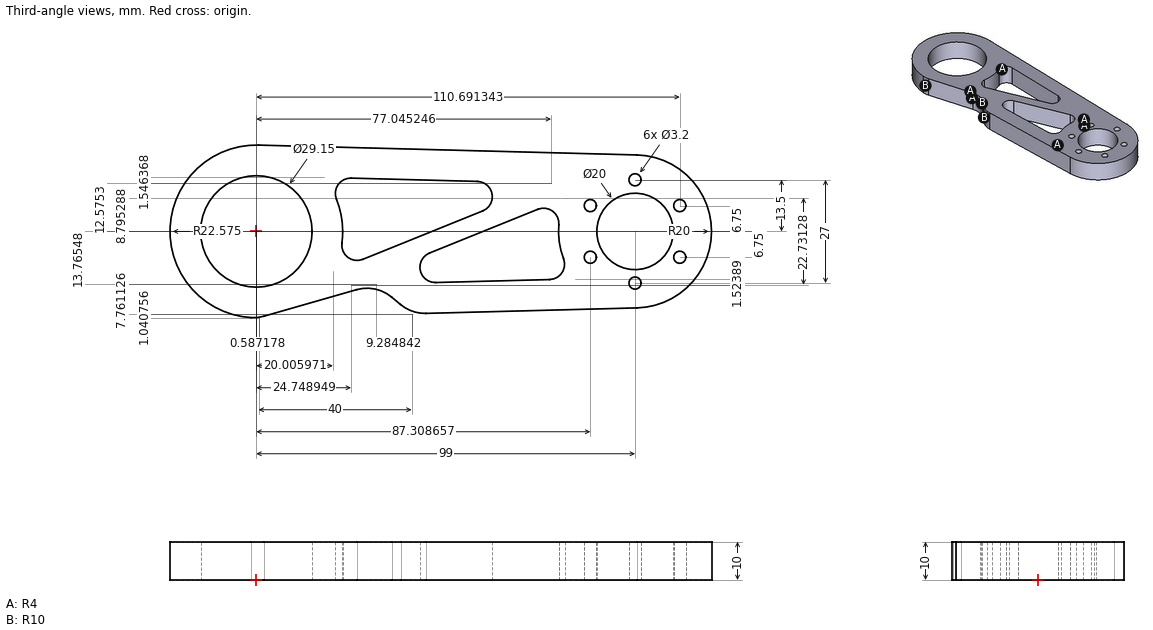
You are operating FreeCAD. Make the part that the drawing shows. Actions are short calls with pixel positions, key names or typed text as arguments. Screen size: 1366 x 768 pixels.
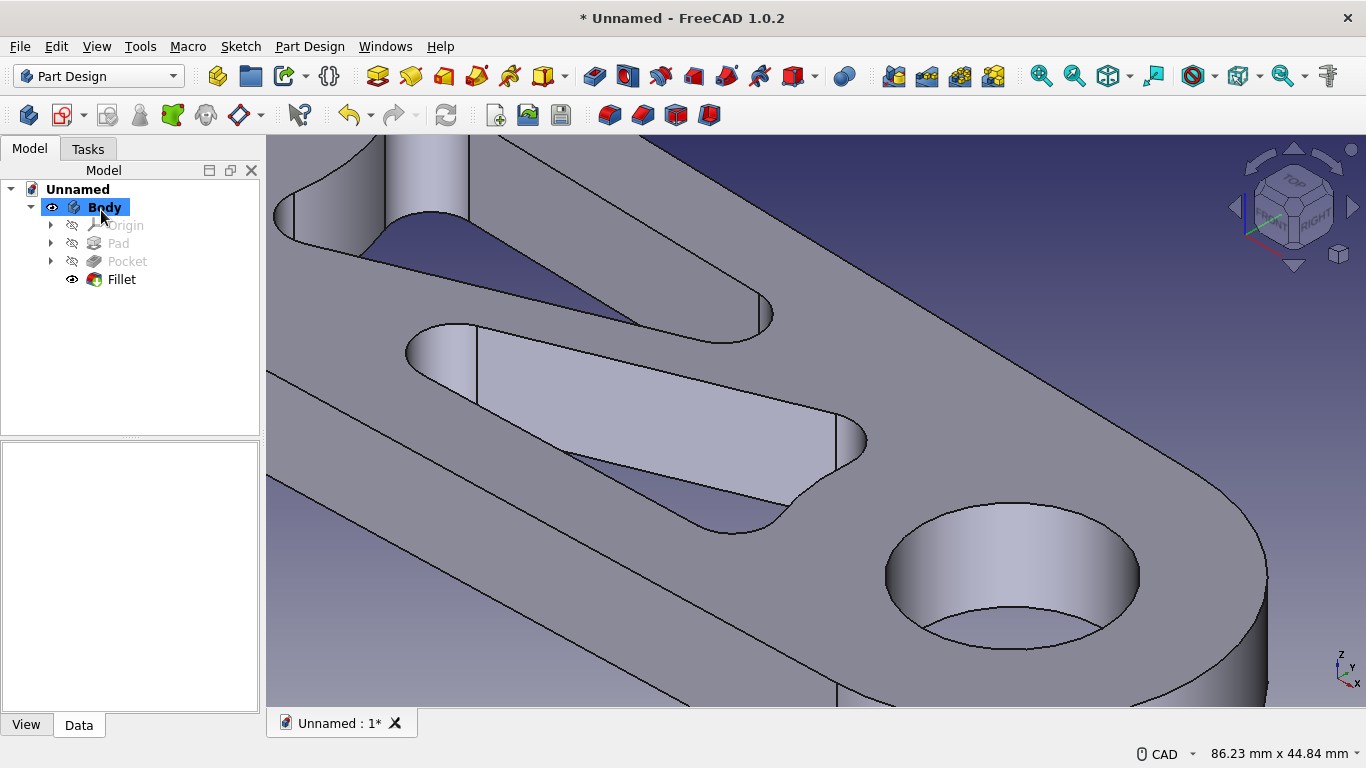
key(v)
key(f)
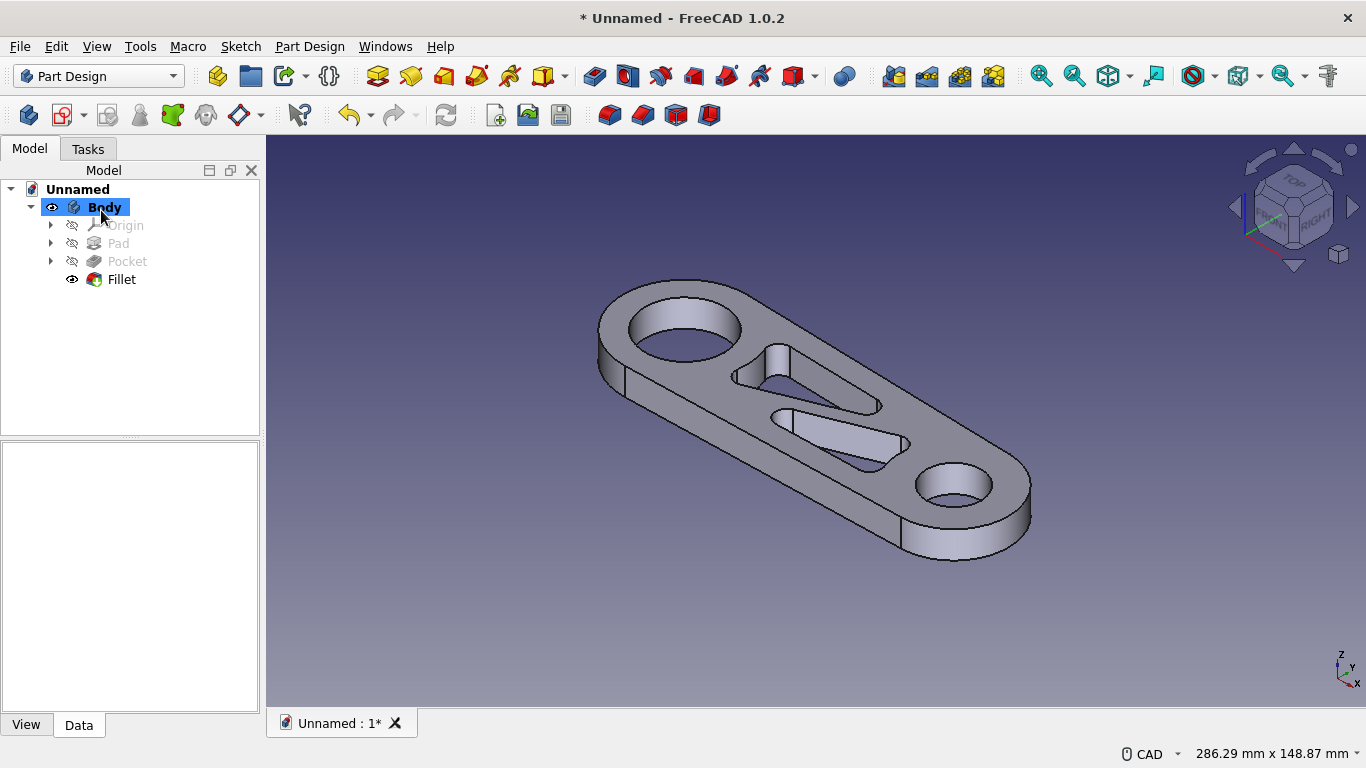
click(906, 416)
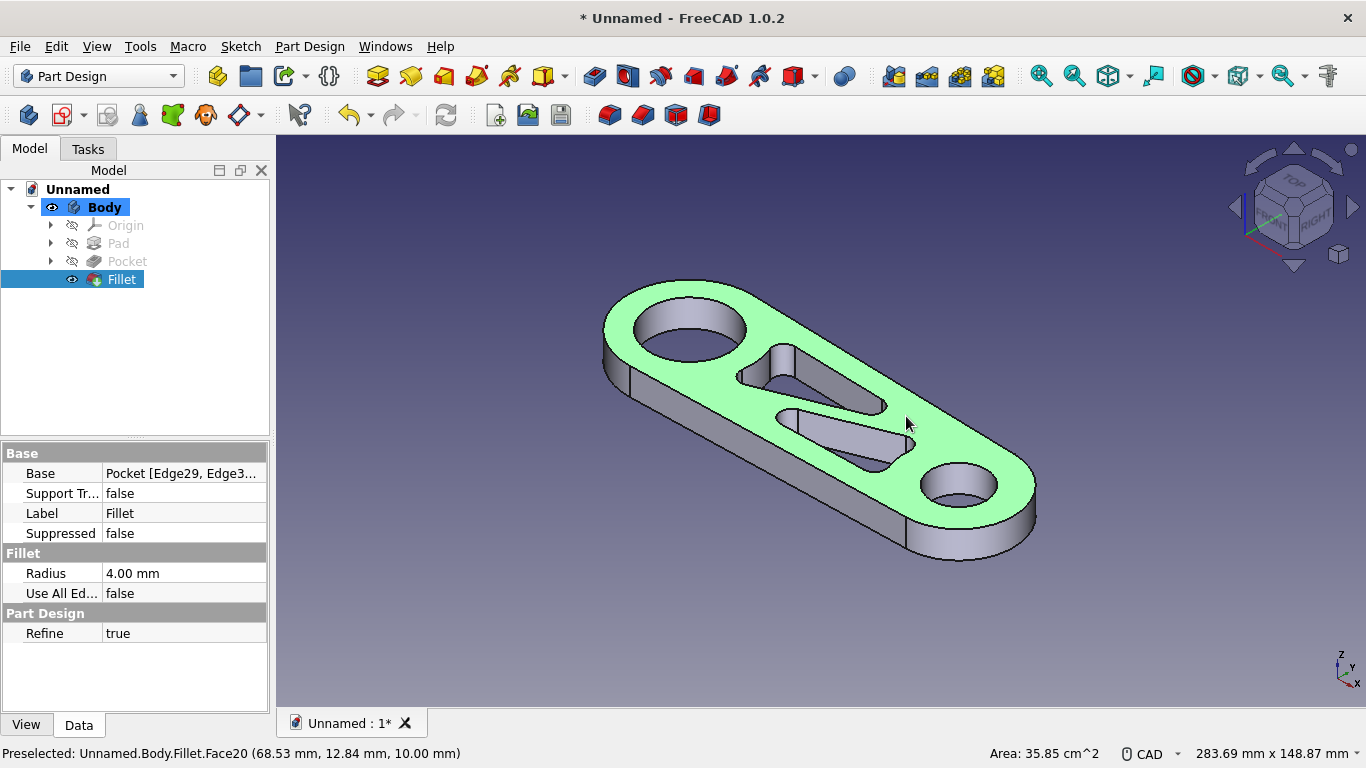
click(62, 116)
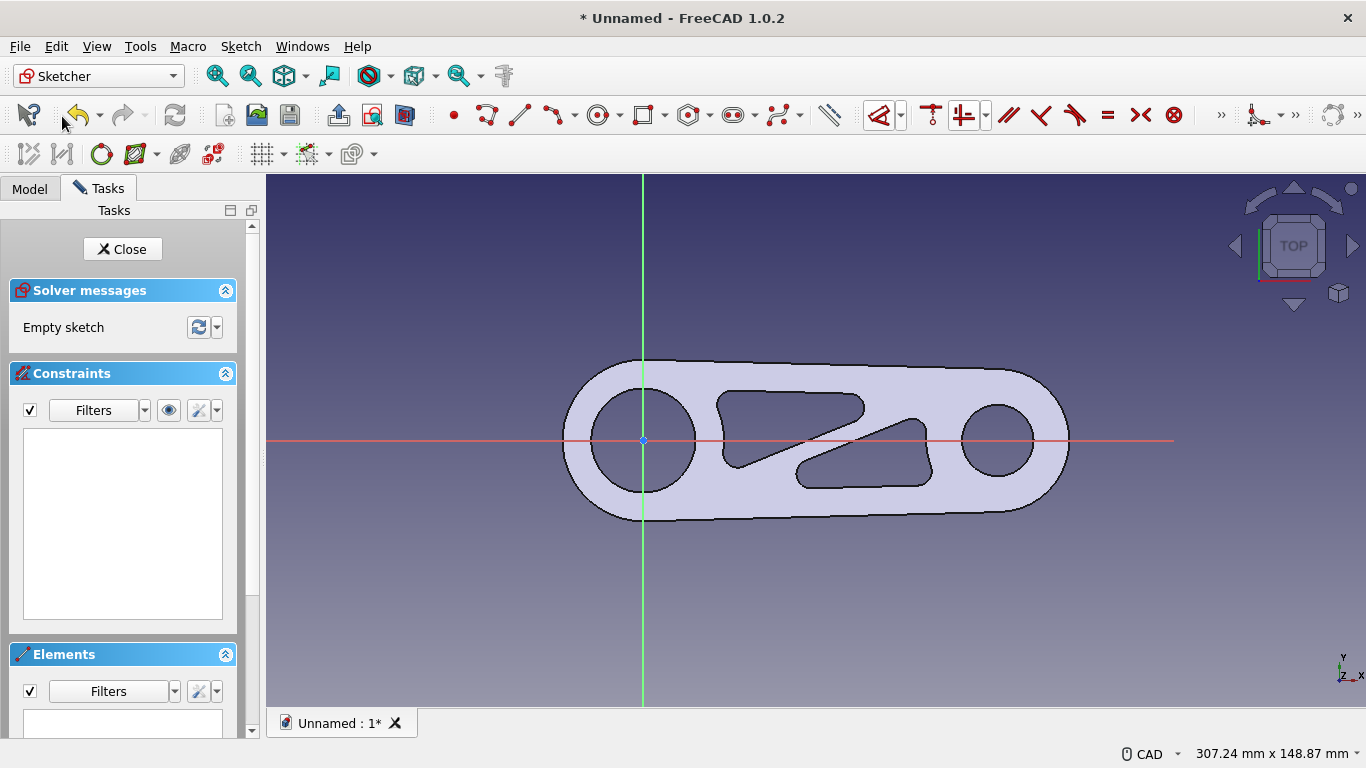
scroll(1106, 440, up, 6)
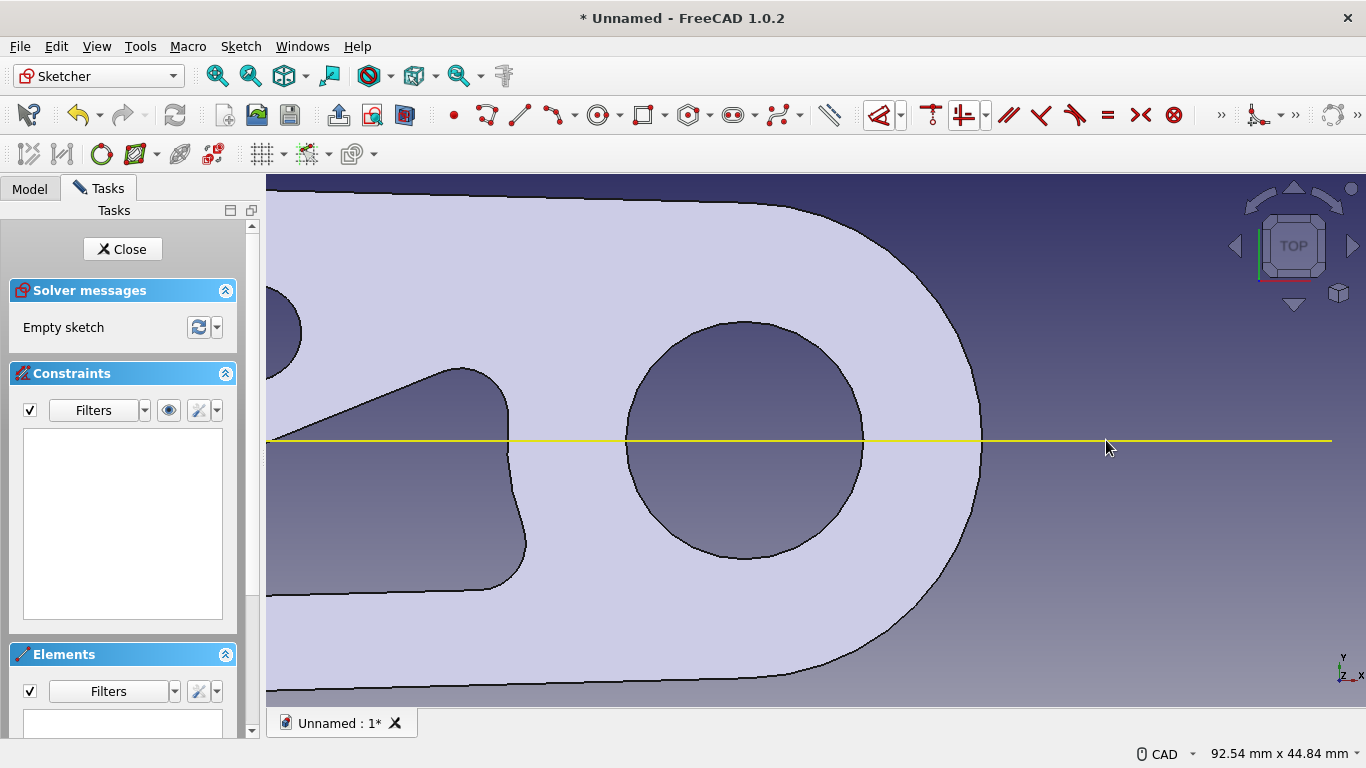
click(598, 116)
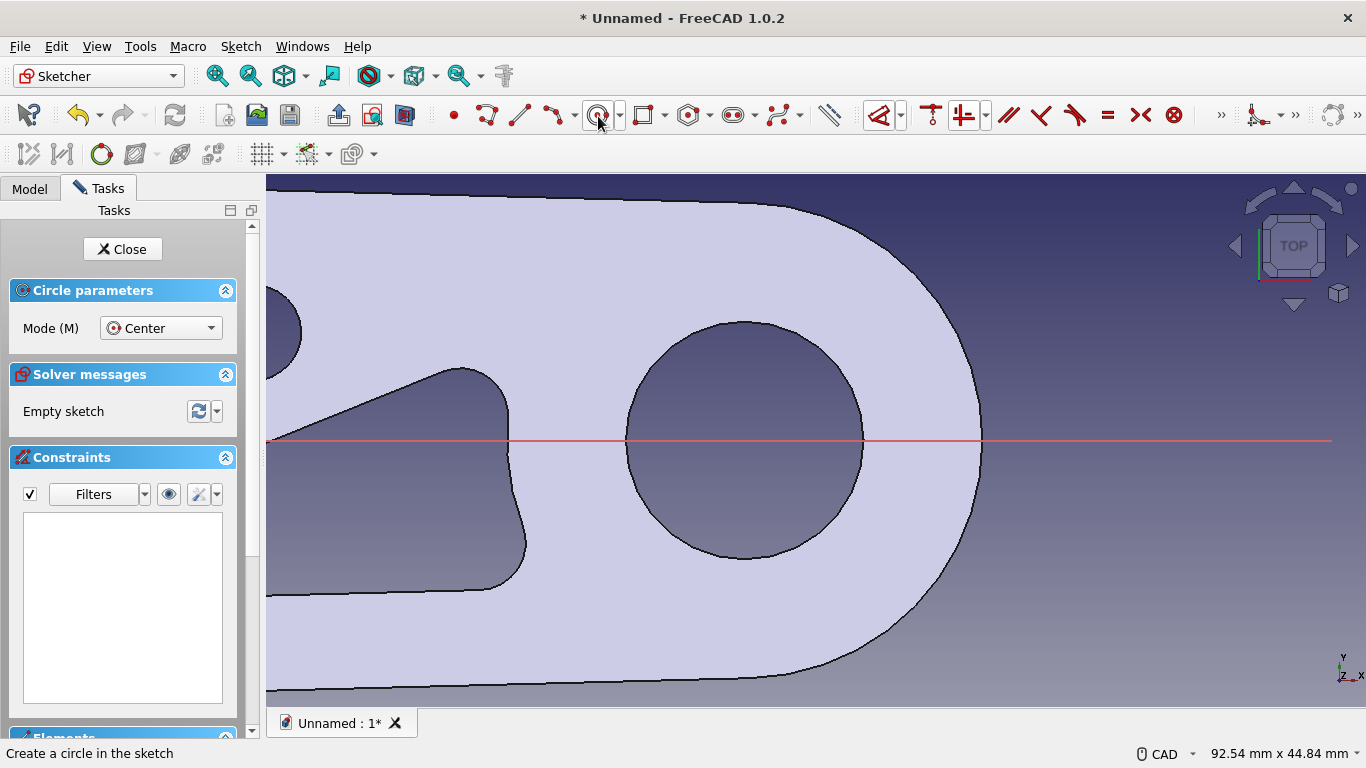
click(745, 280)
move(758, 267)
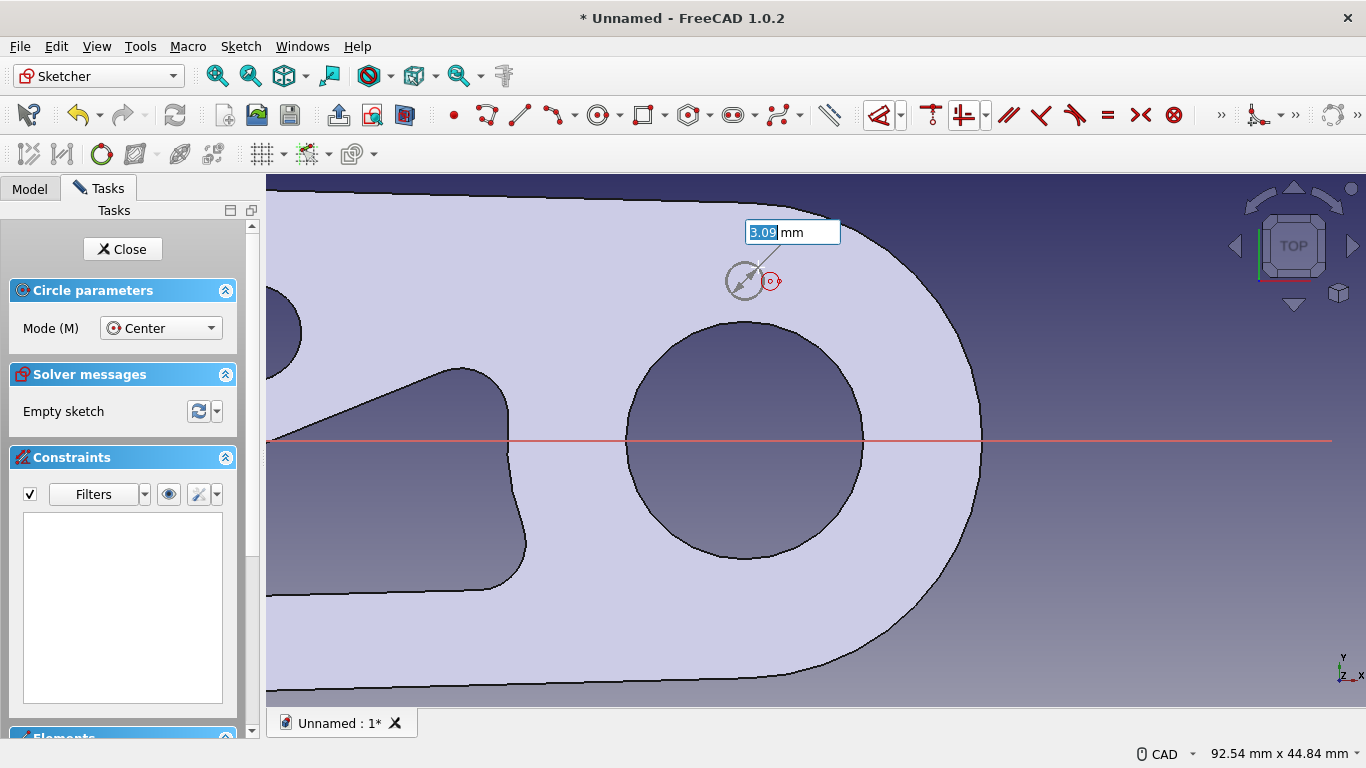
text(3.2)
key(Return)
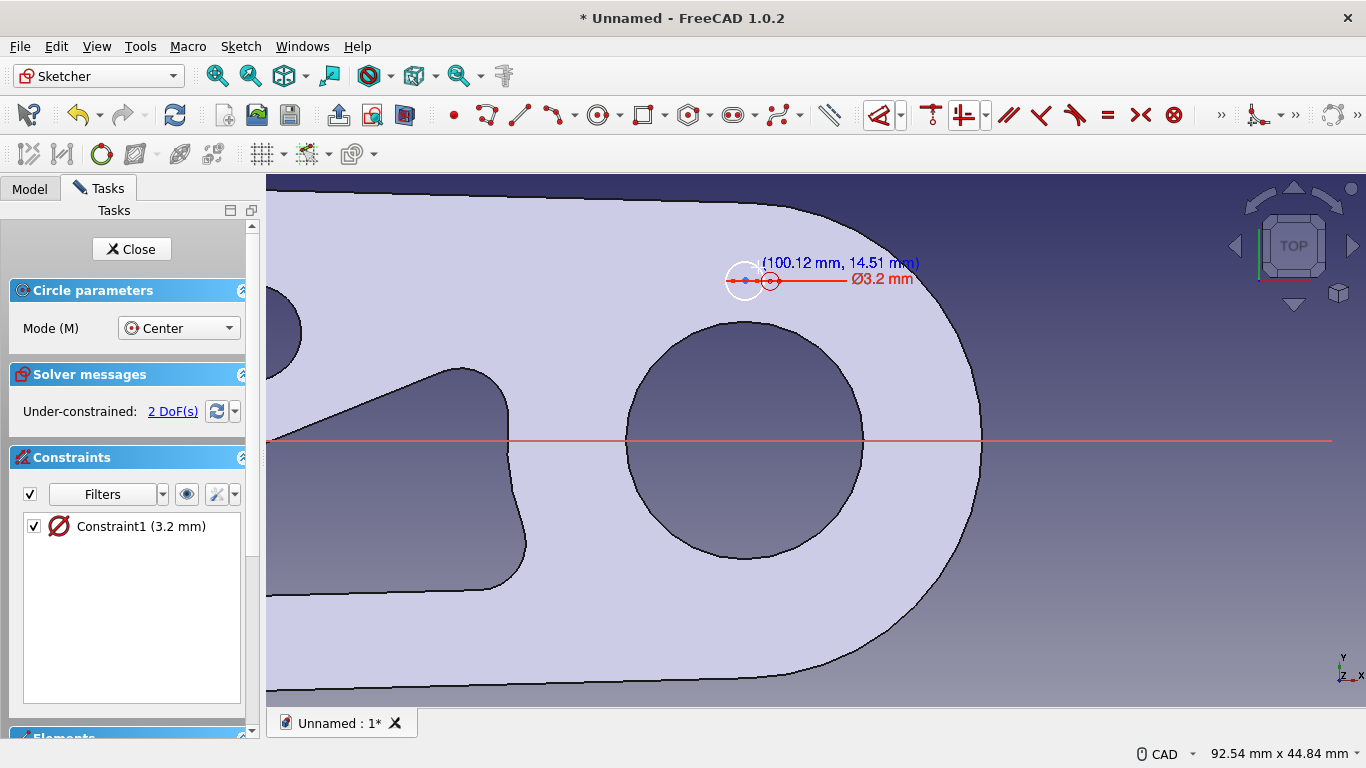
click(884, 360)
move(897, 347)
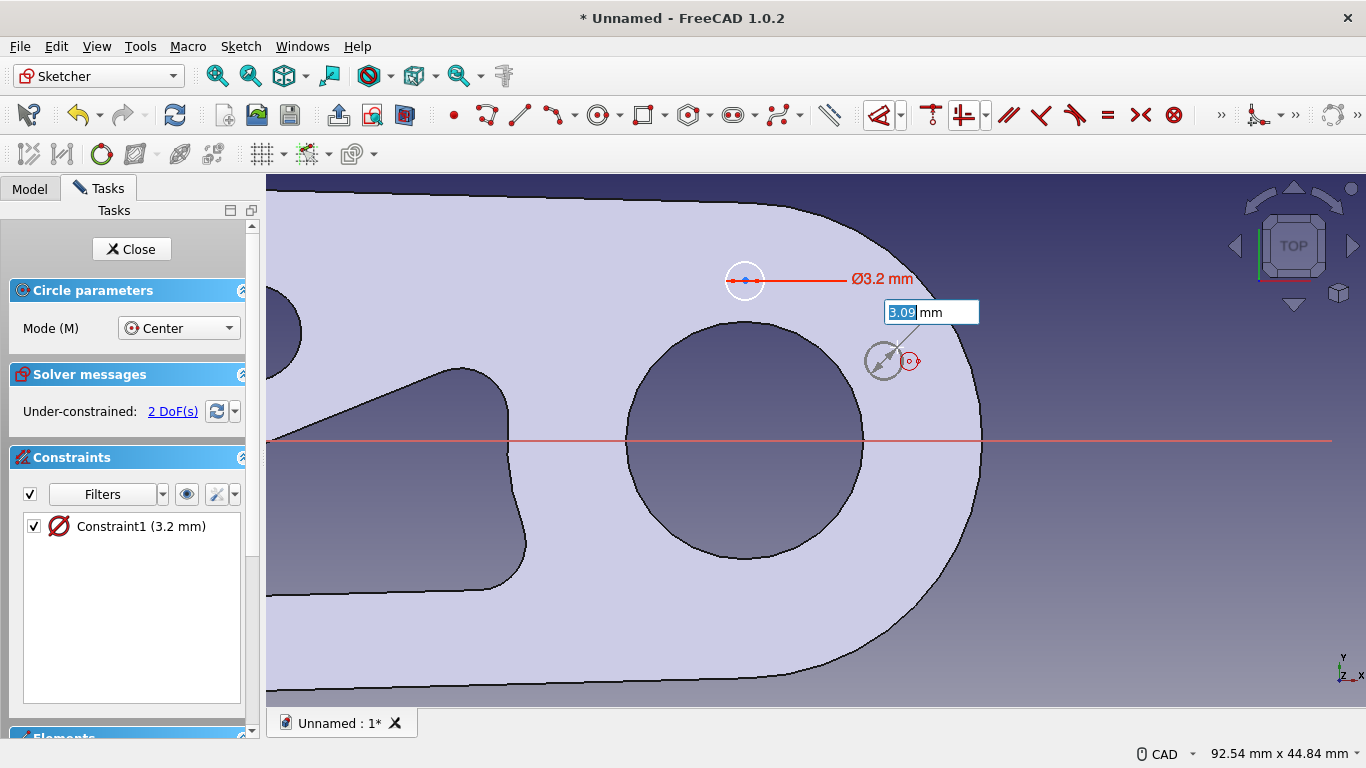
text(3.2)
key(Return)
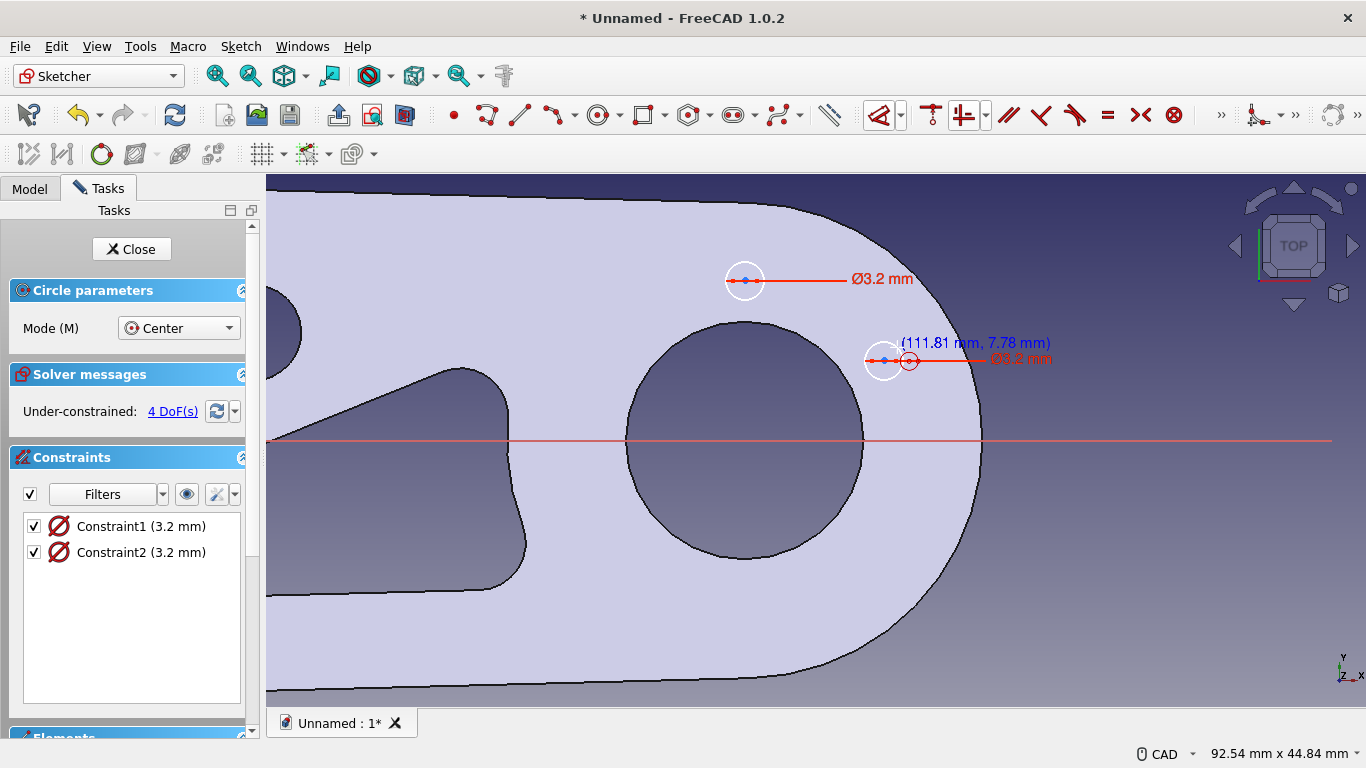
click(884, 521)
move(897, 507)